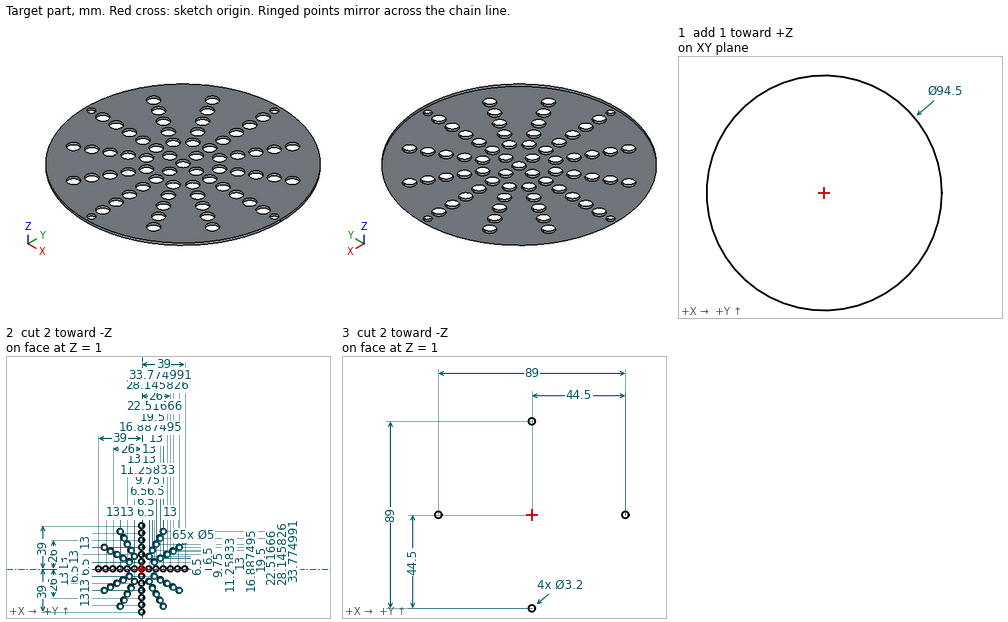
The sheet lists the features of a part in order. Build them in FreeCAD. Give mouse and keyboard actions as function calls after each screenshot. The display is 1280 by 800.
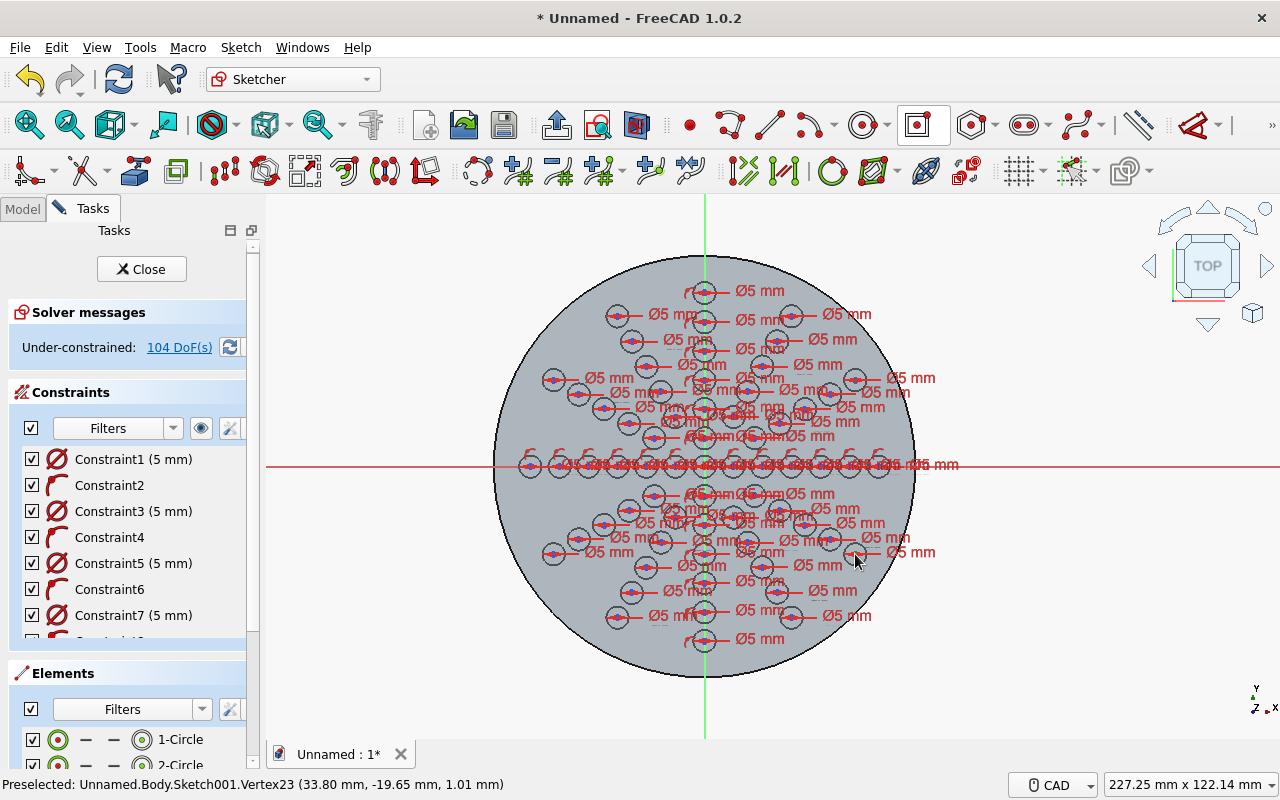
click(353, 467)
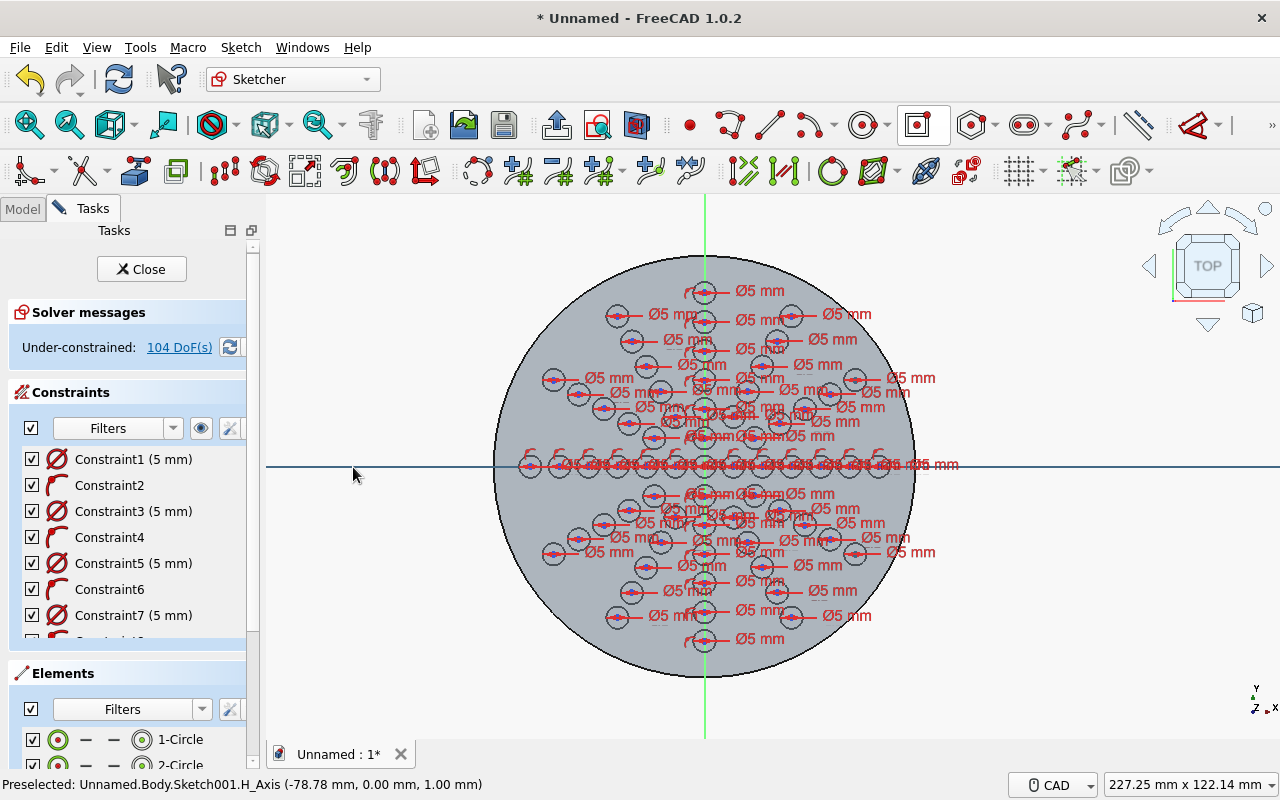
key(s)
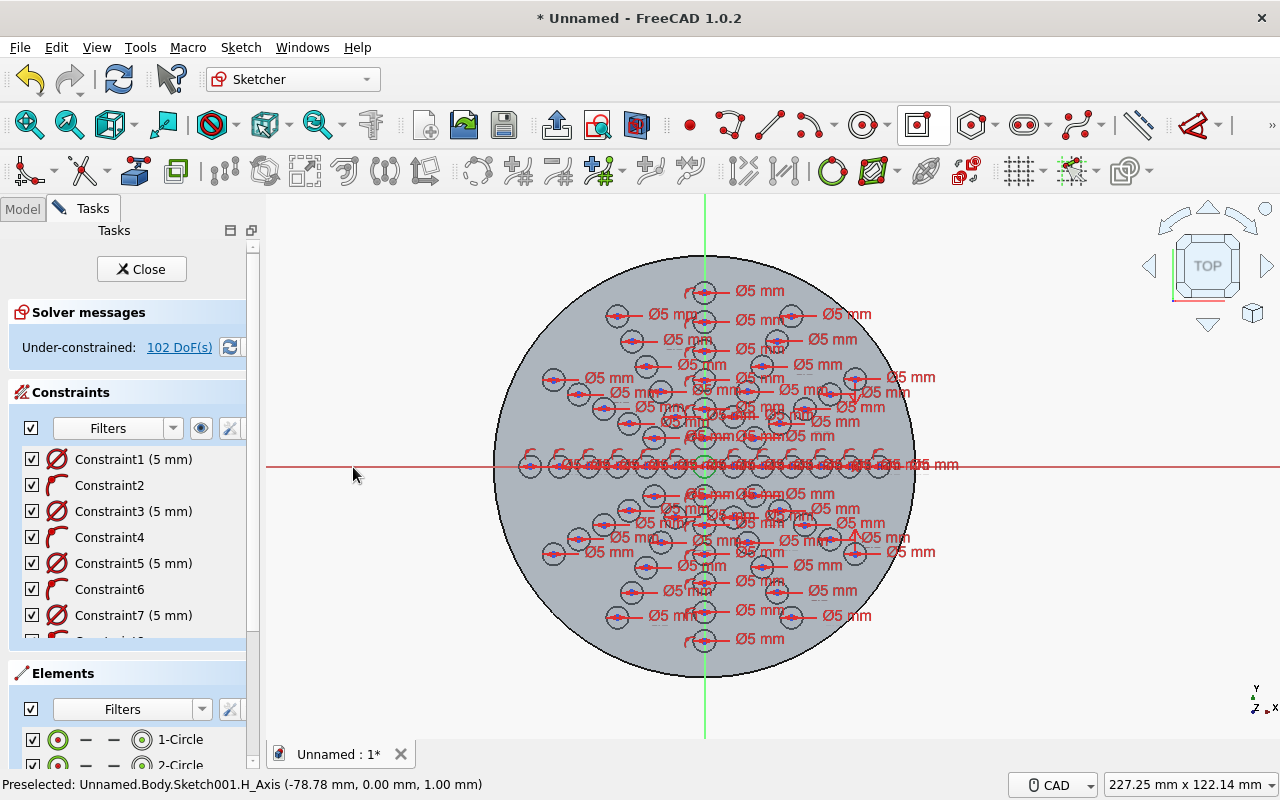
click(830, 394)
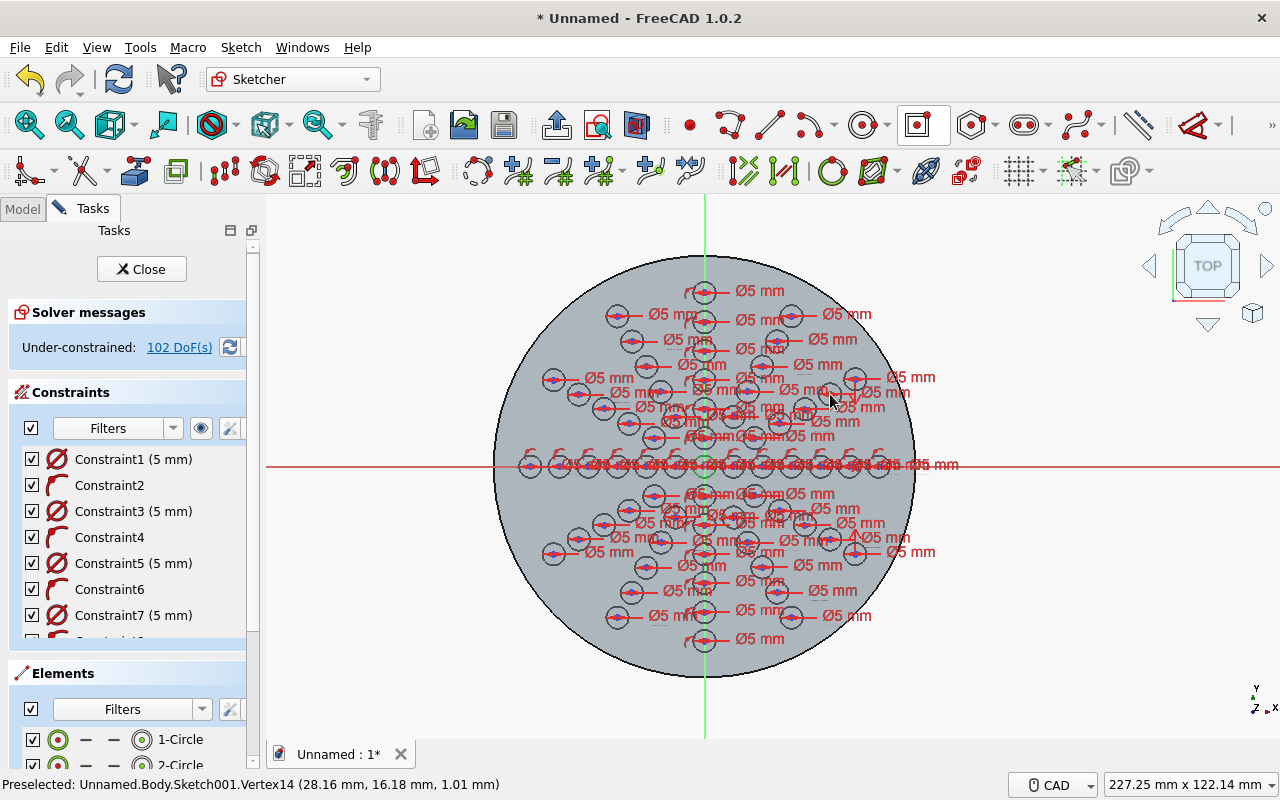
click(830, 540)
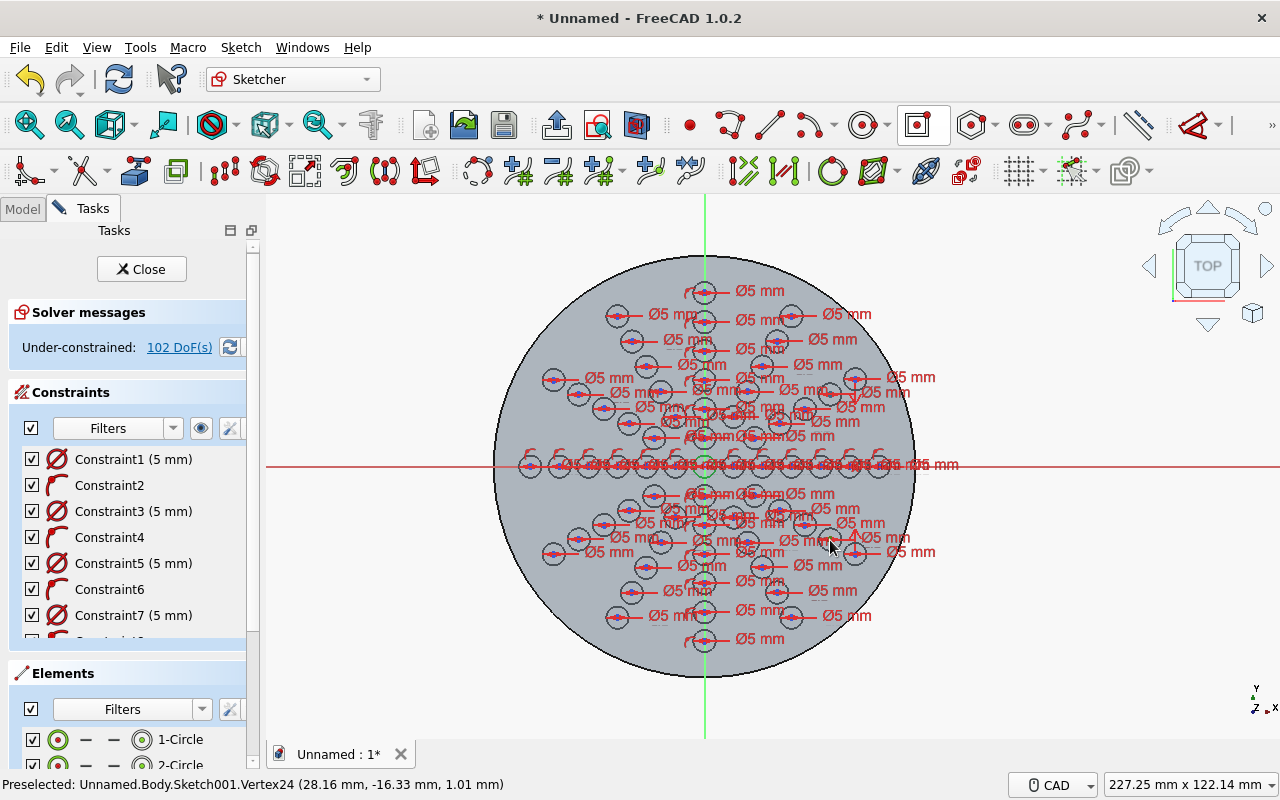
click(353, 467)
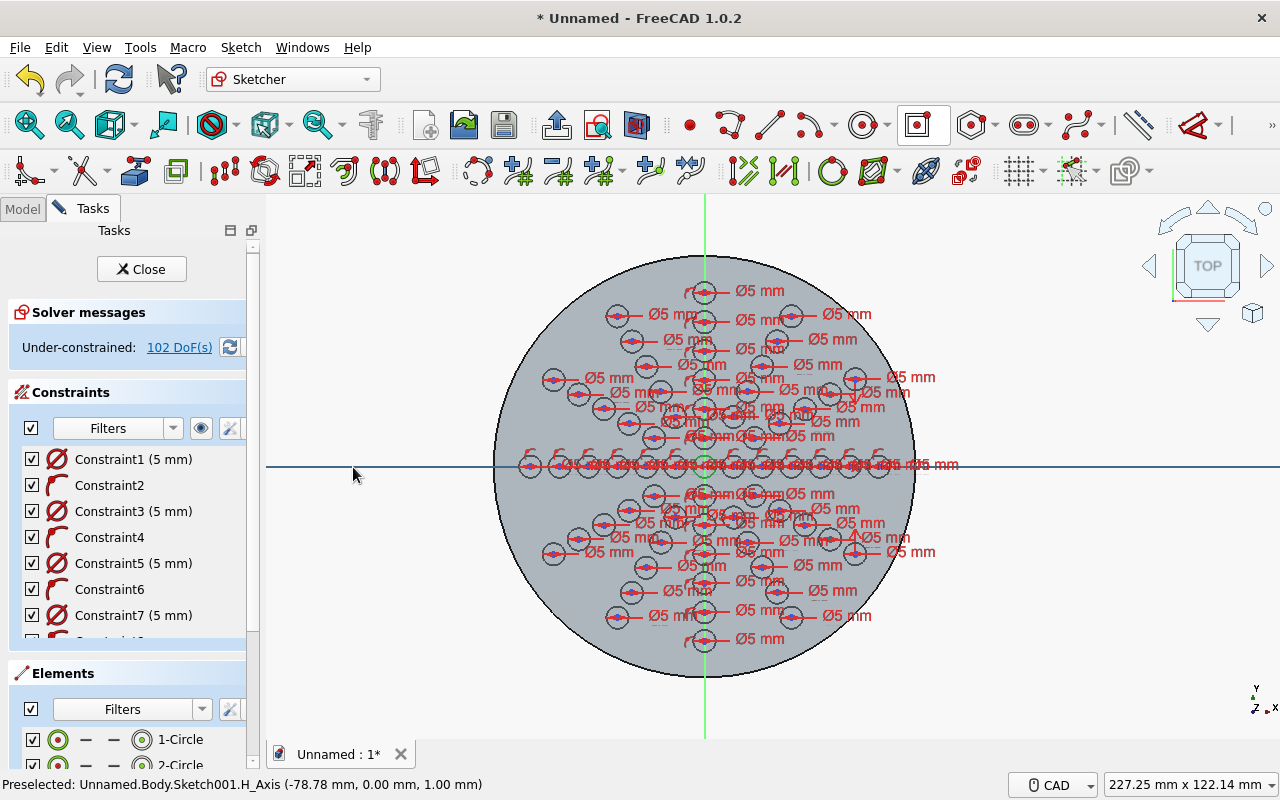
key(s)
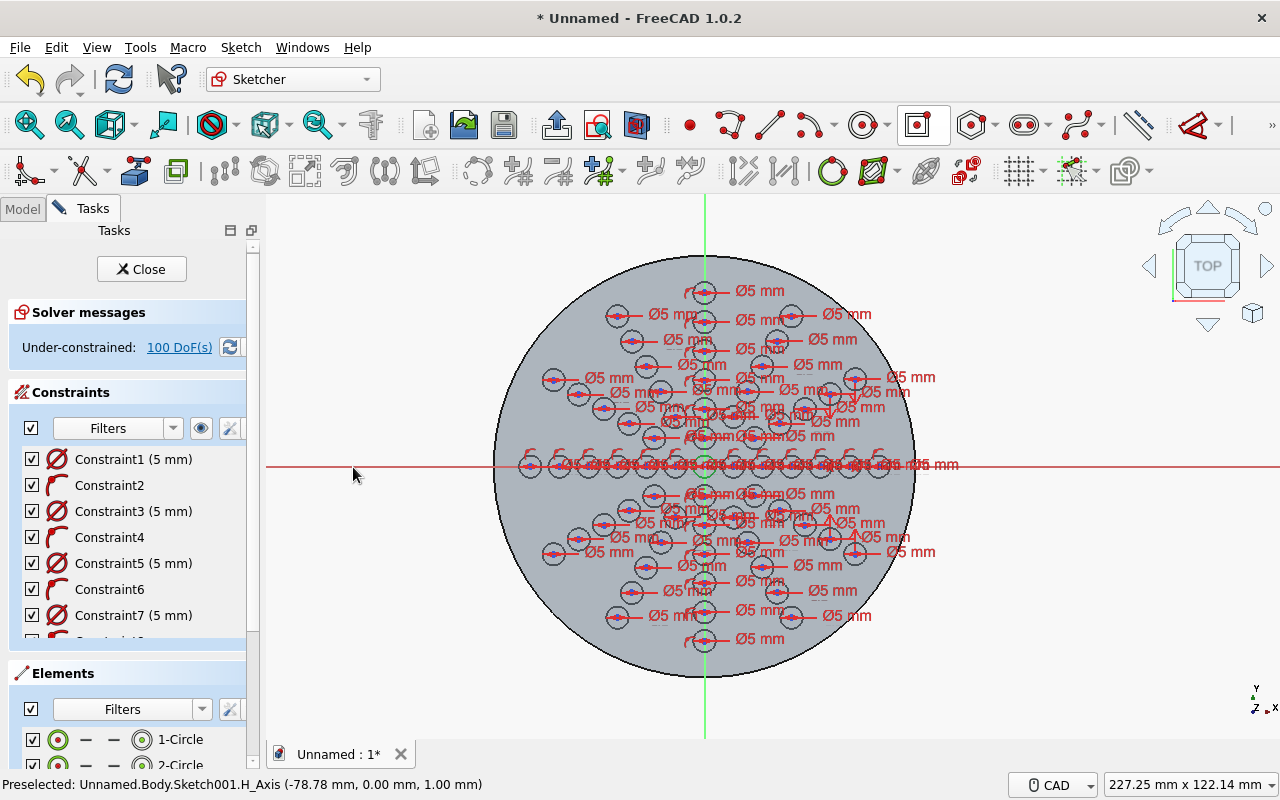
click(805, 409)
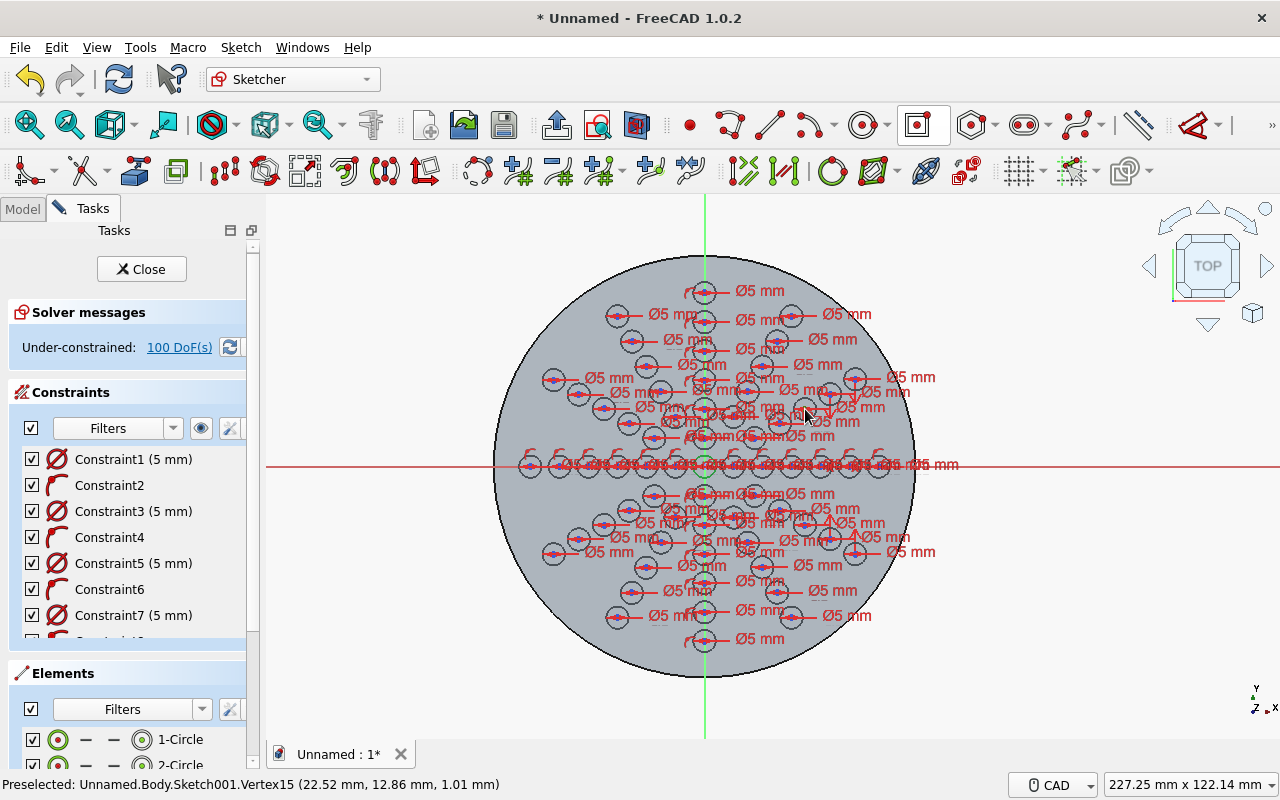
click(805, 525)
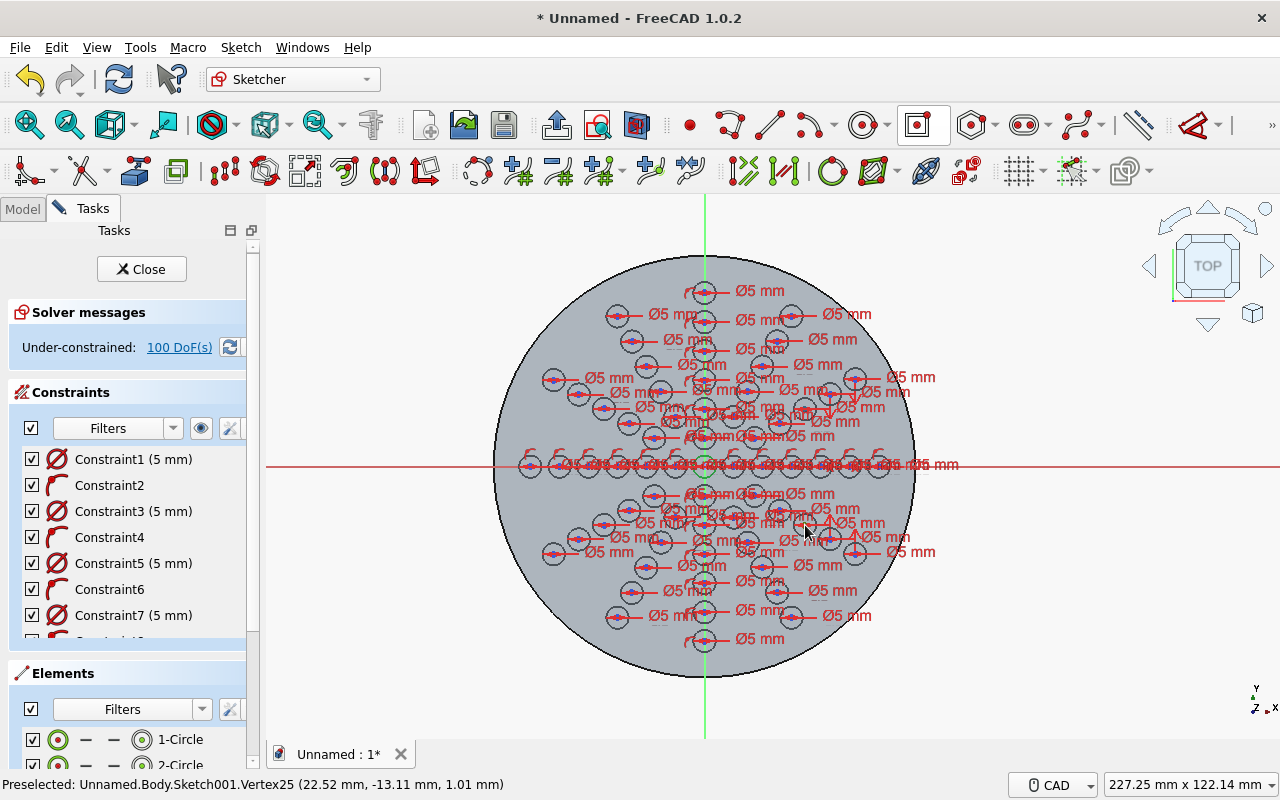
click(353, 467)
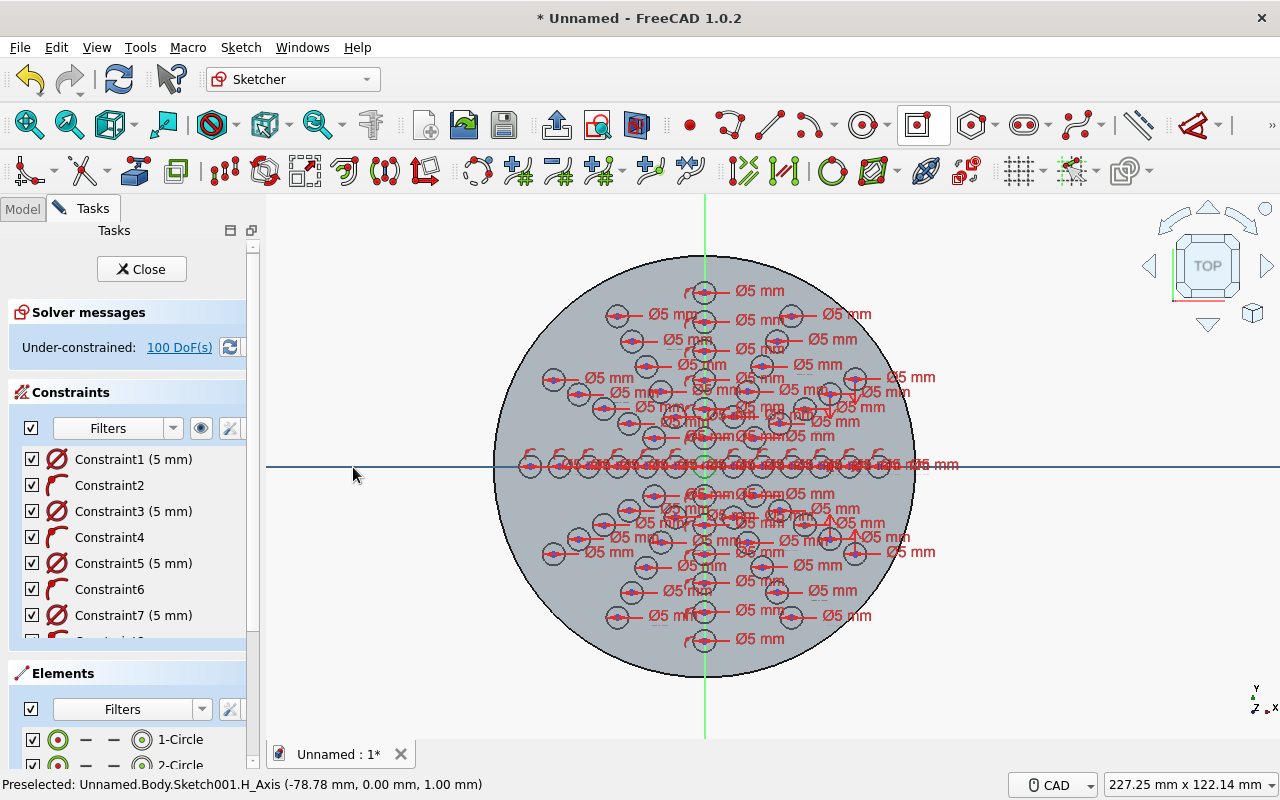
key(s)